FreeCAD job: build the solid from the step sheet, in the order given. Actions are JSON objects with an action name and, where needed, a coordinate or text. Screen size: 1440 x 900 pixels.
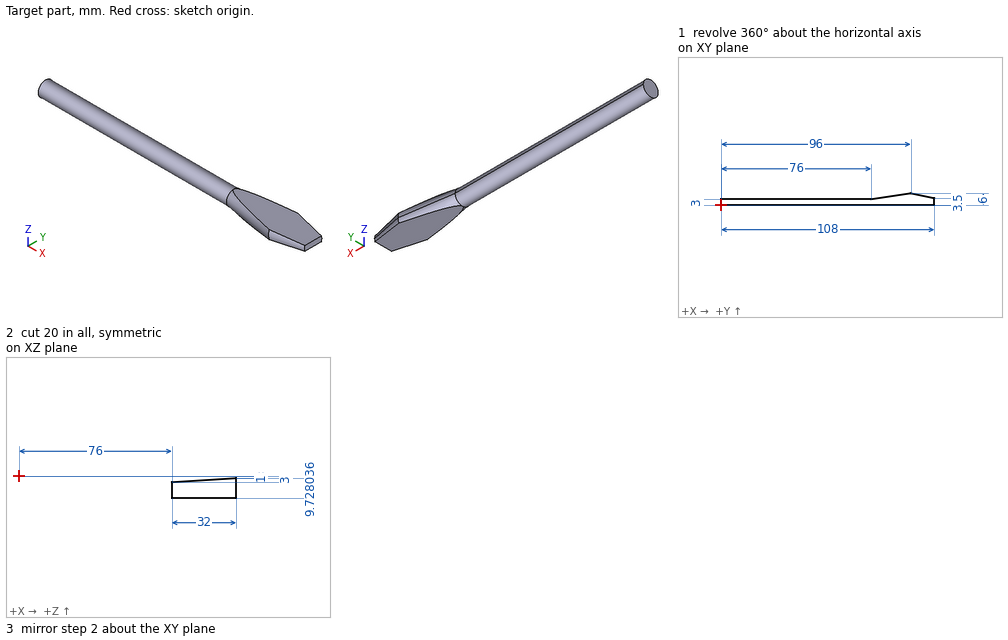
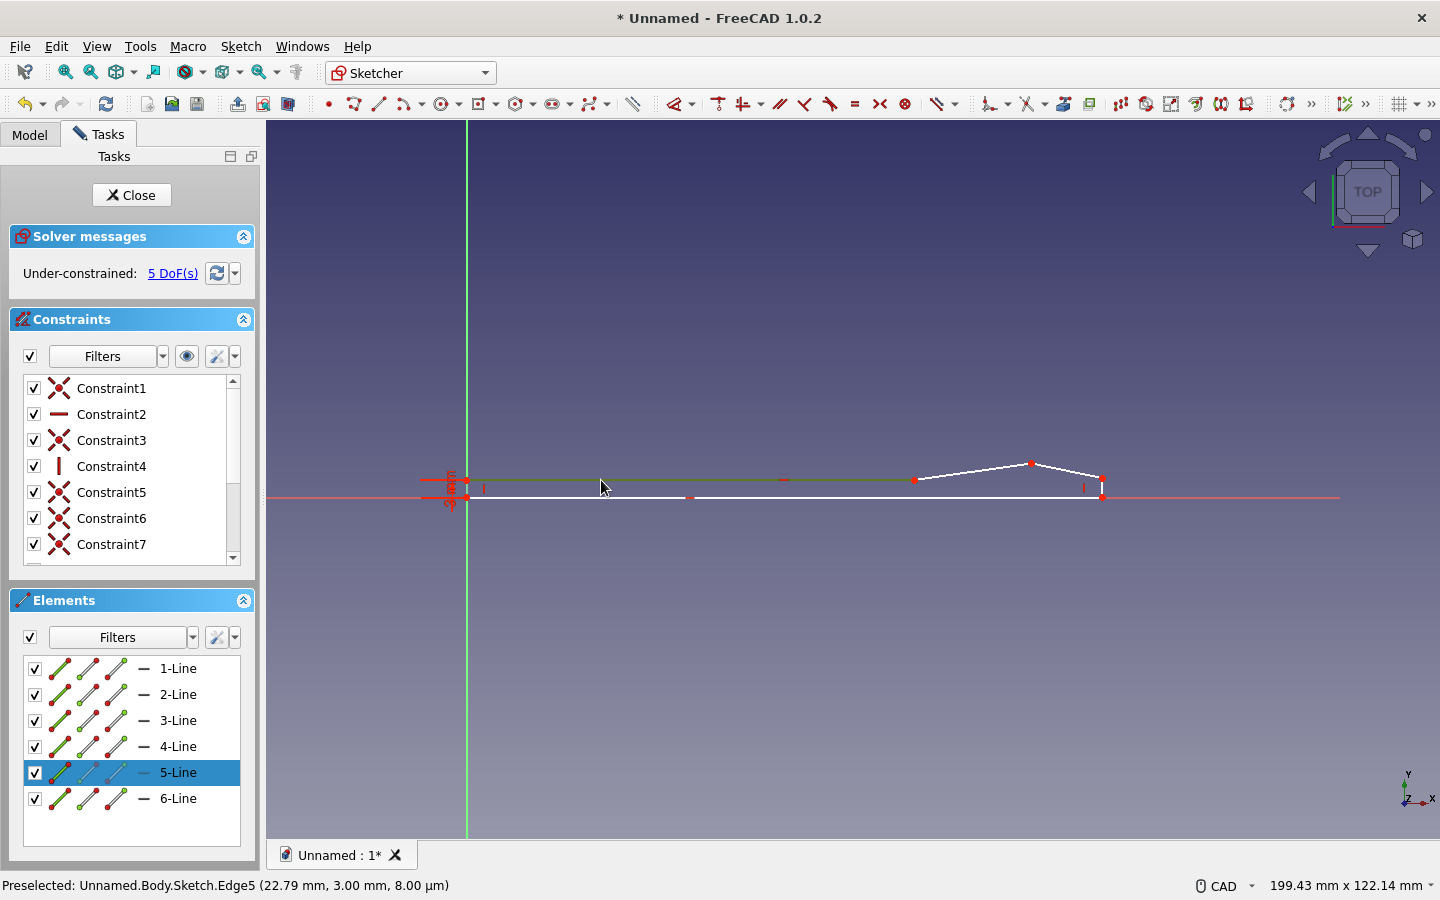
{"action": "key", "text": "l"}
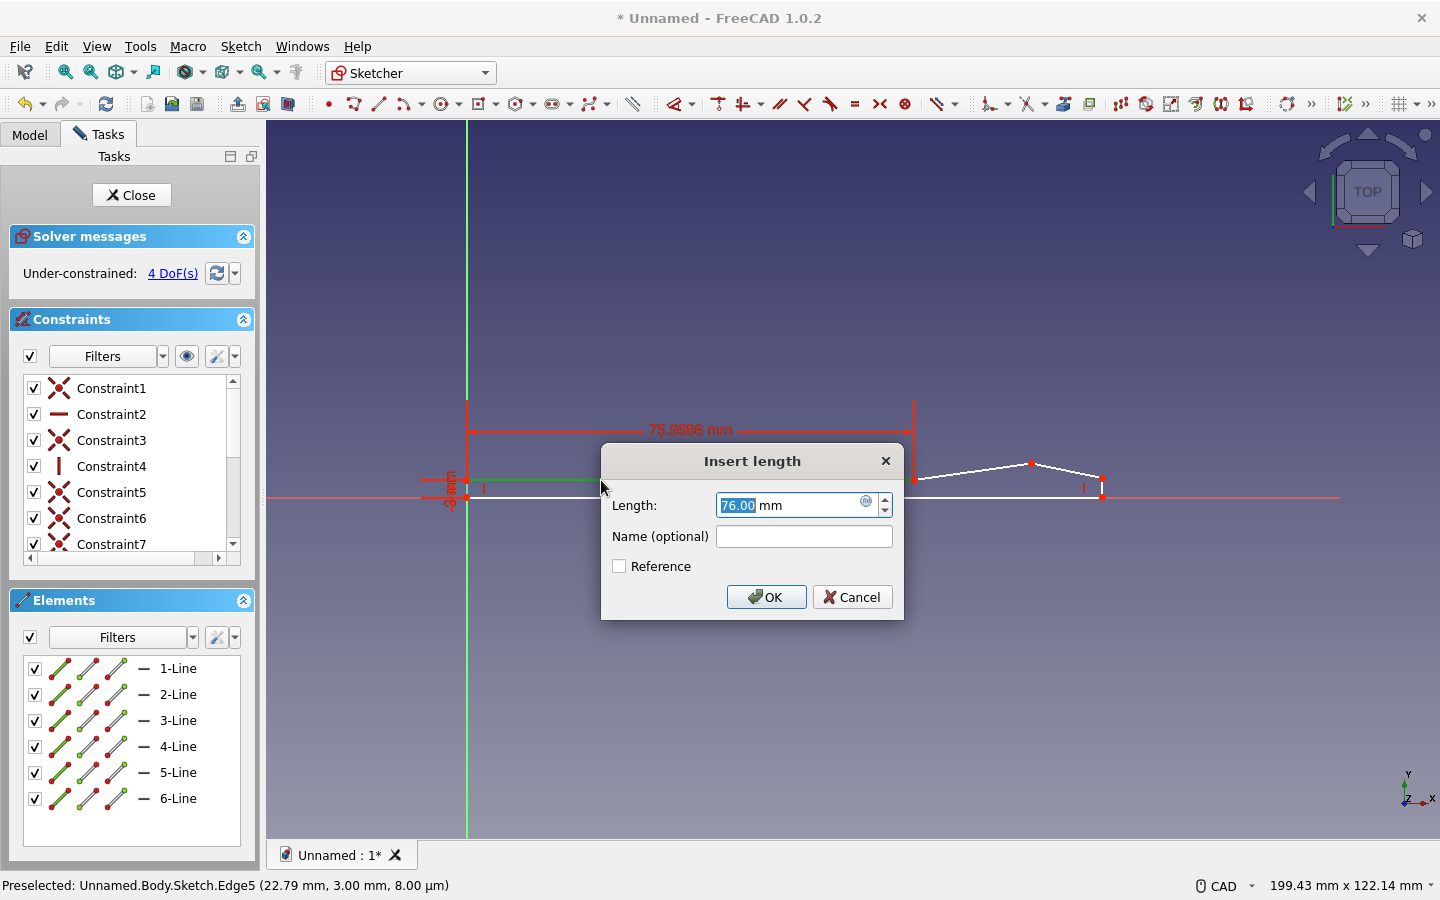
{"action": "type", "text": "76"}
{"action": "key", "text": "Return"}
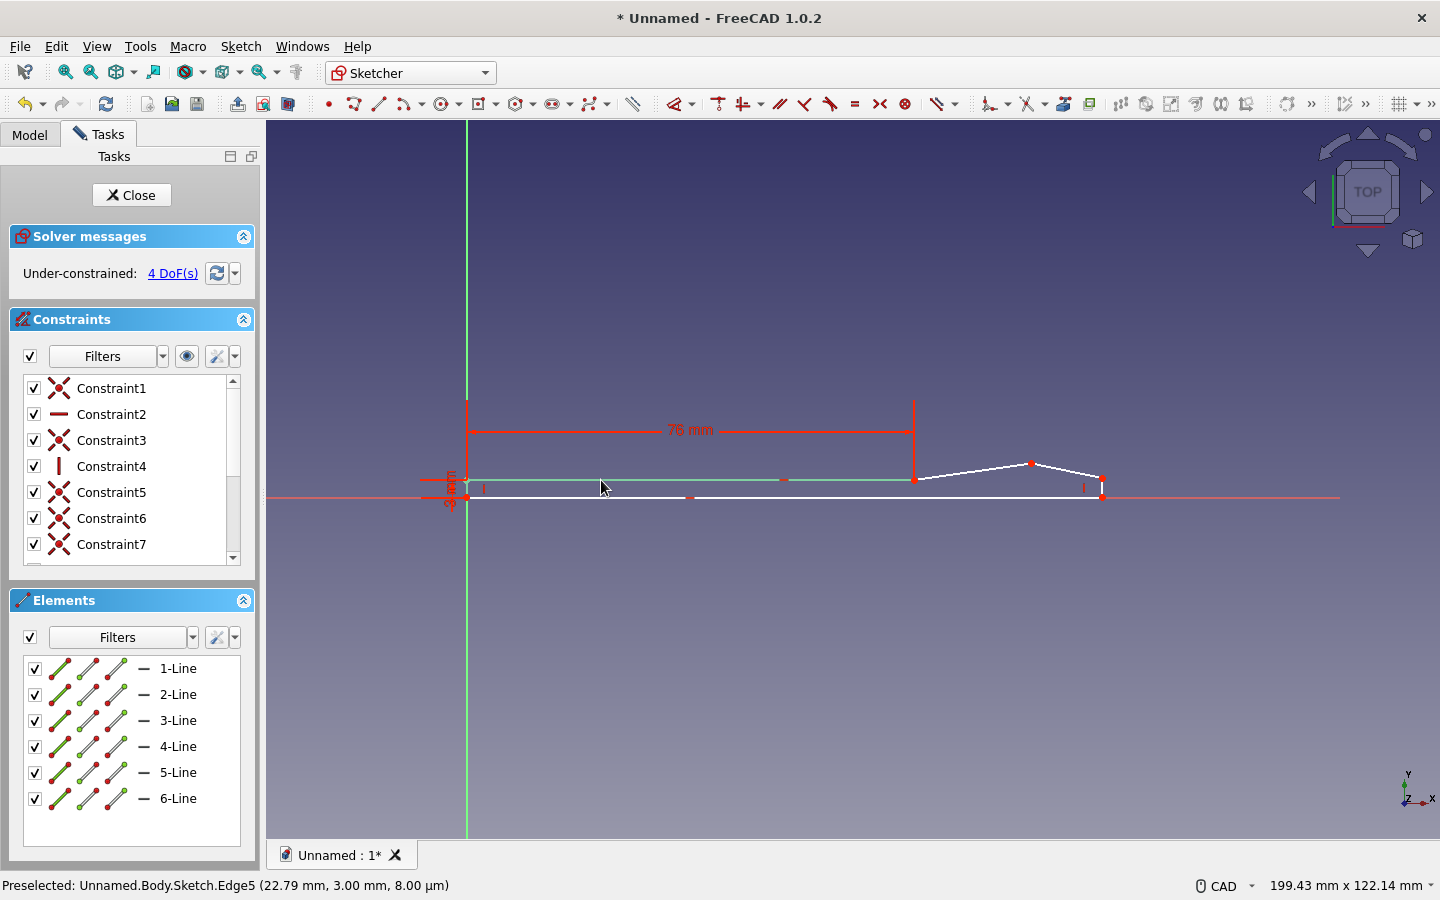
{"action": "left_click", "coordinate": [1032, 463]}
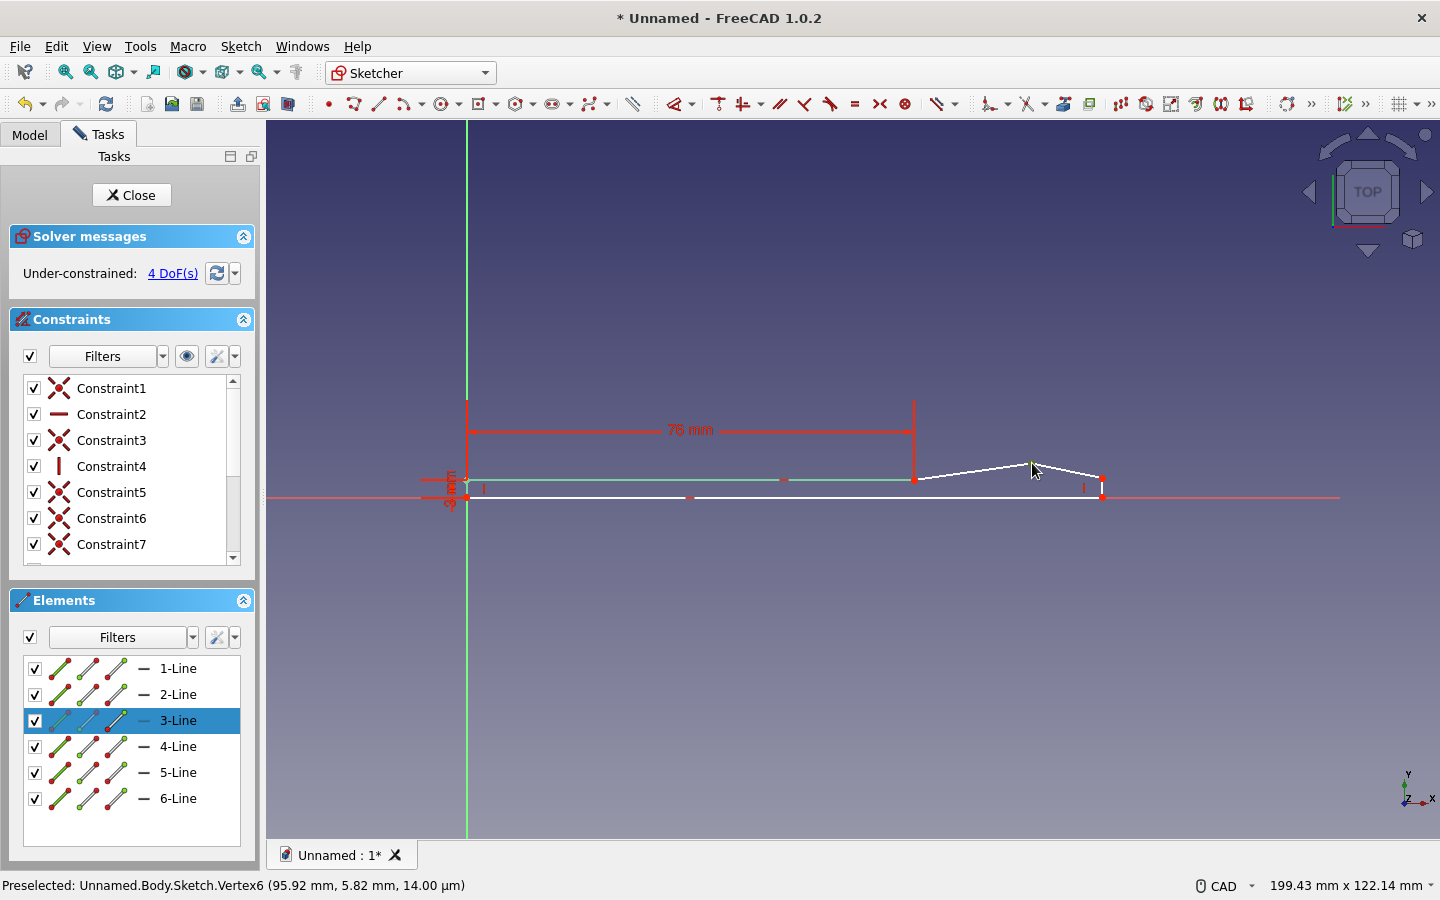
{"action": "key", "text": "i"}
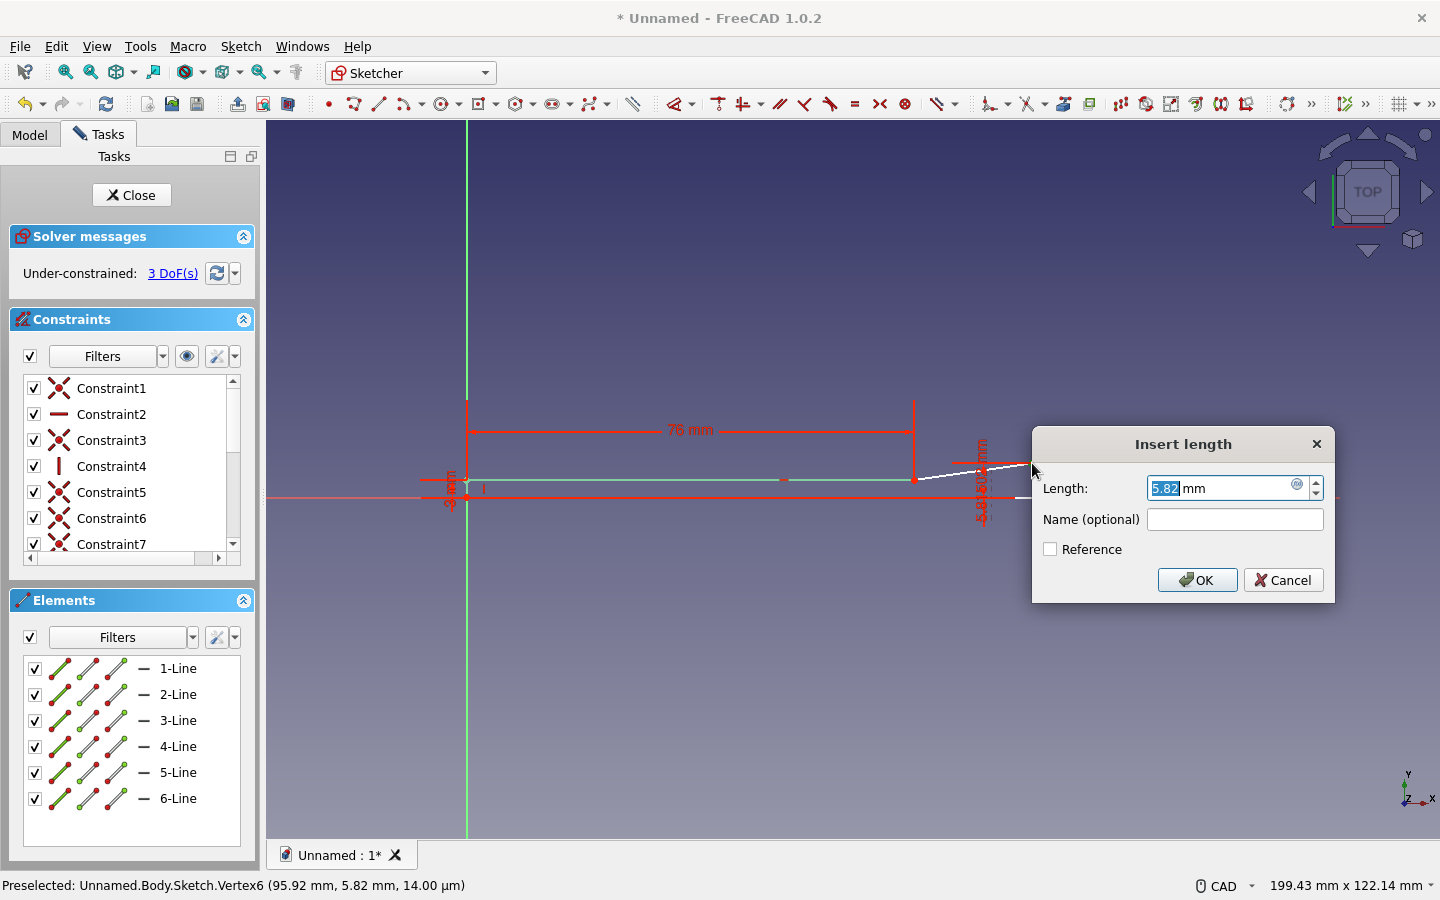
{"action": "type", "text": "6"}
{"action": "key", "text": "Return"}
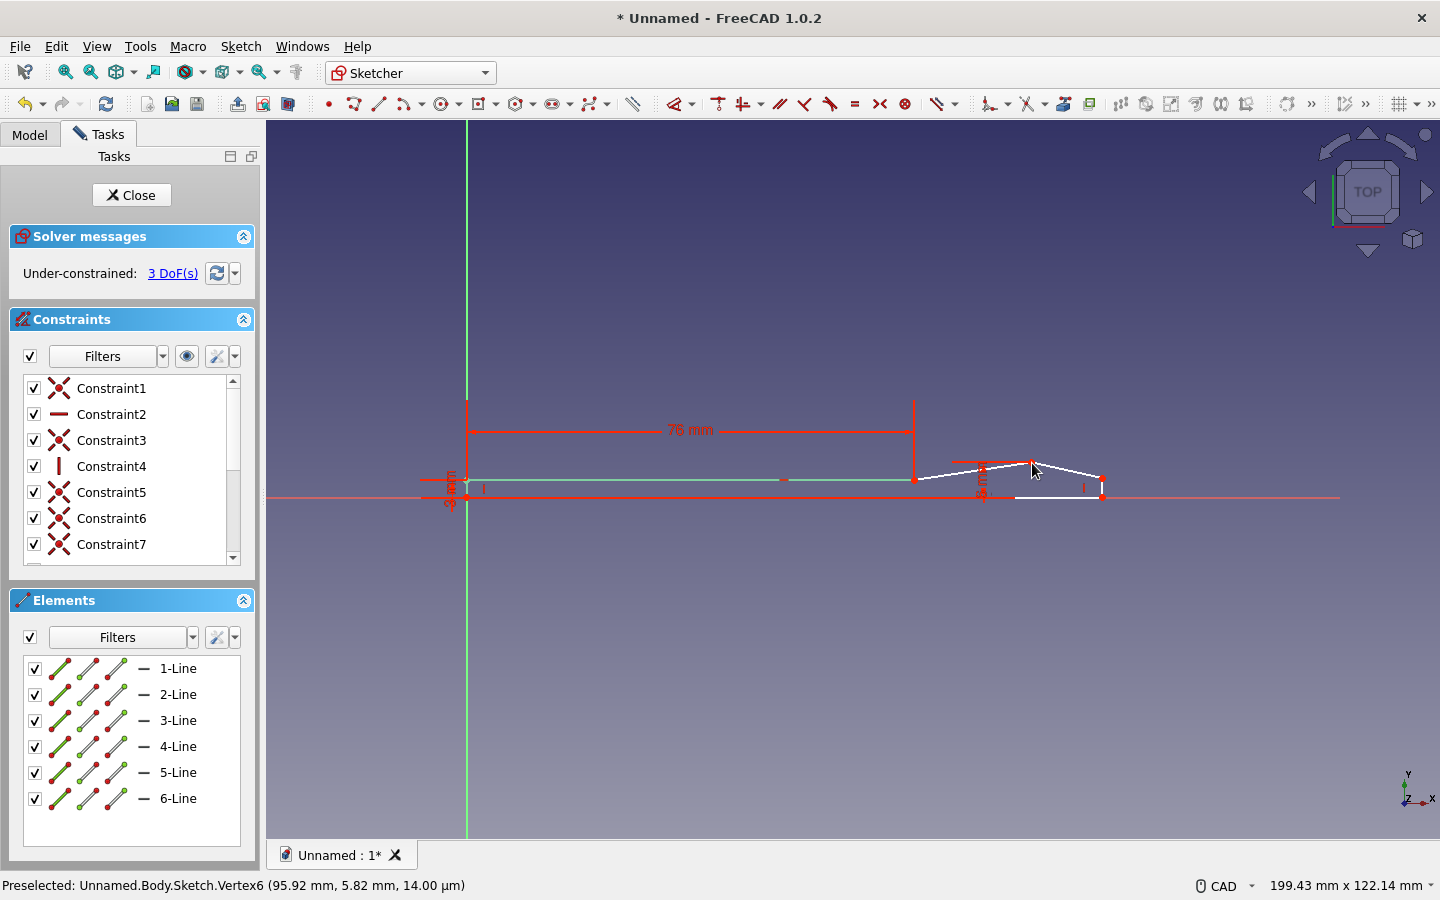
{"action": "left_click", "coordinate": [658, 498]}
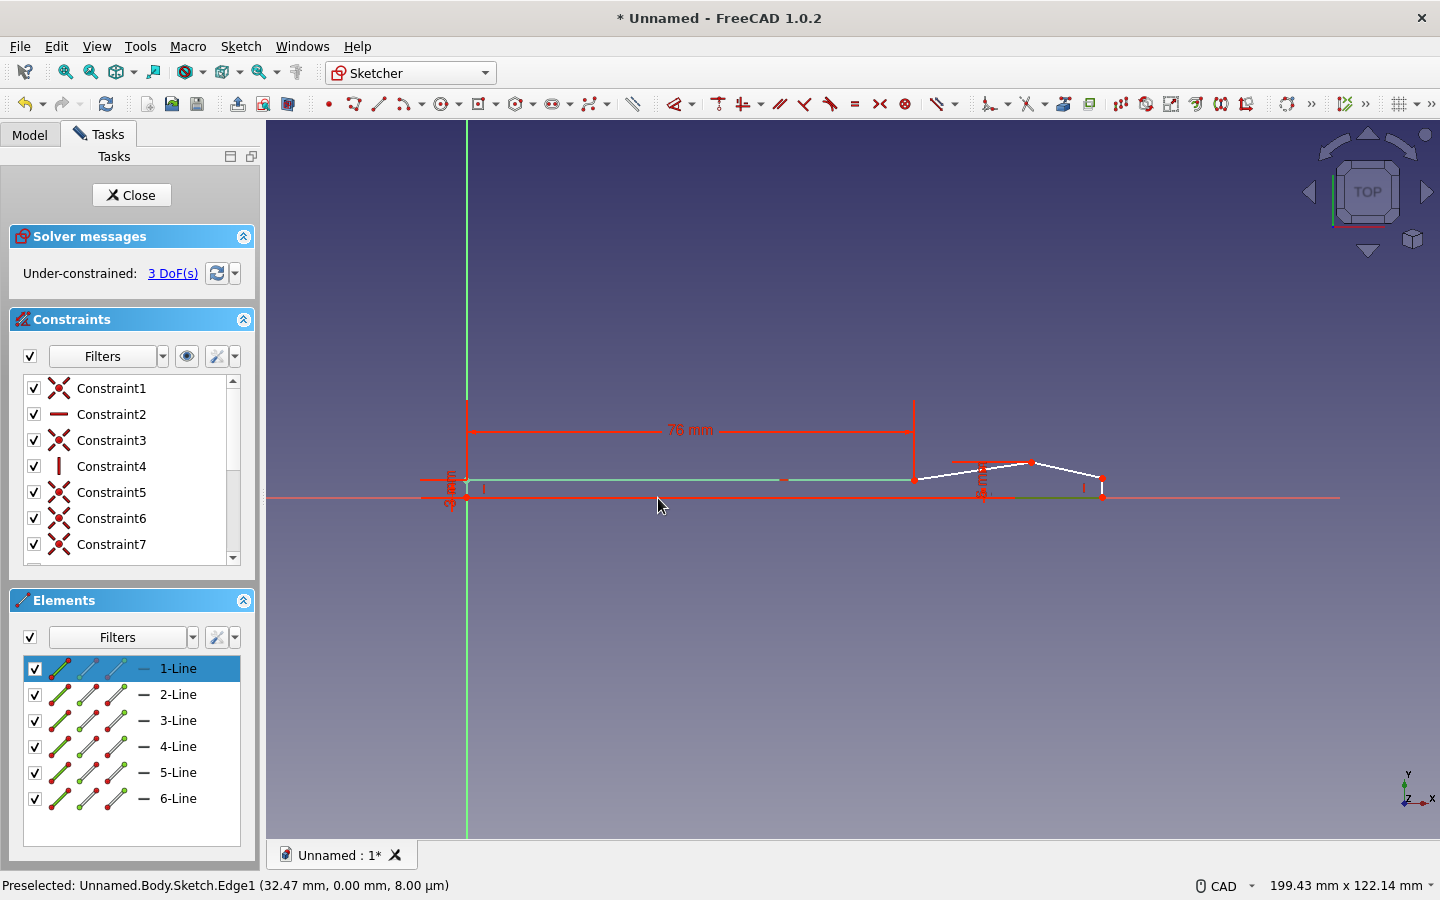
{"action": "left_click", "coordinate": [692, 104]}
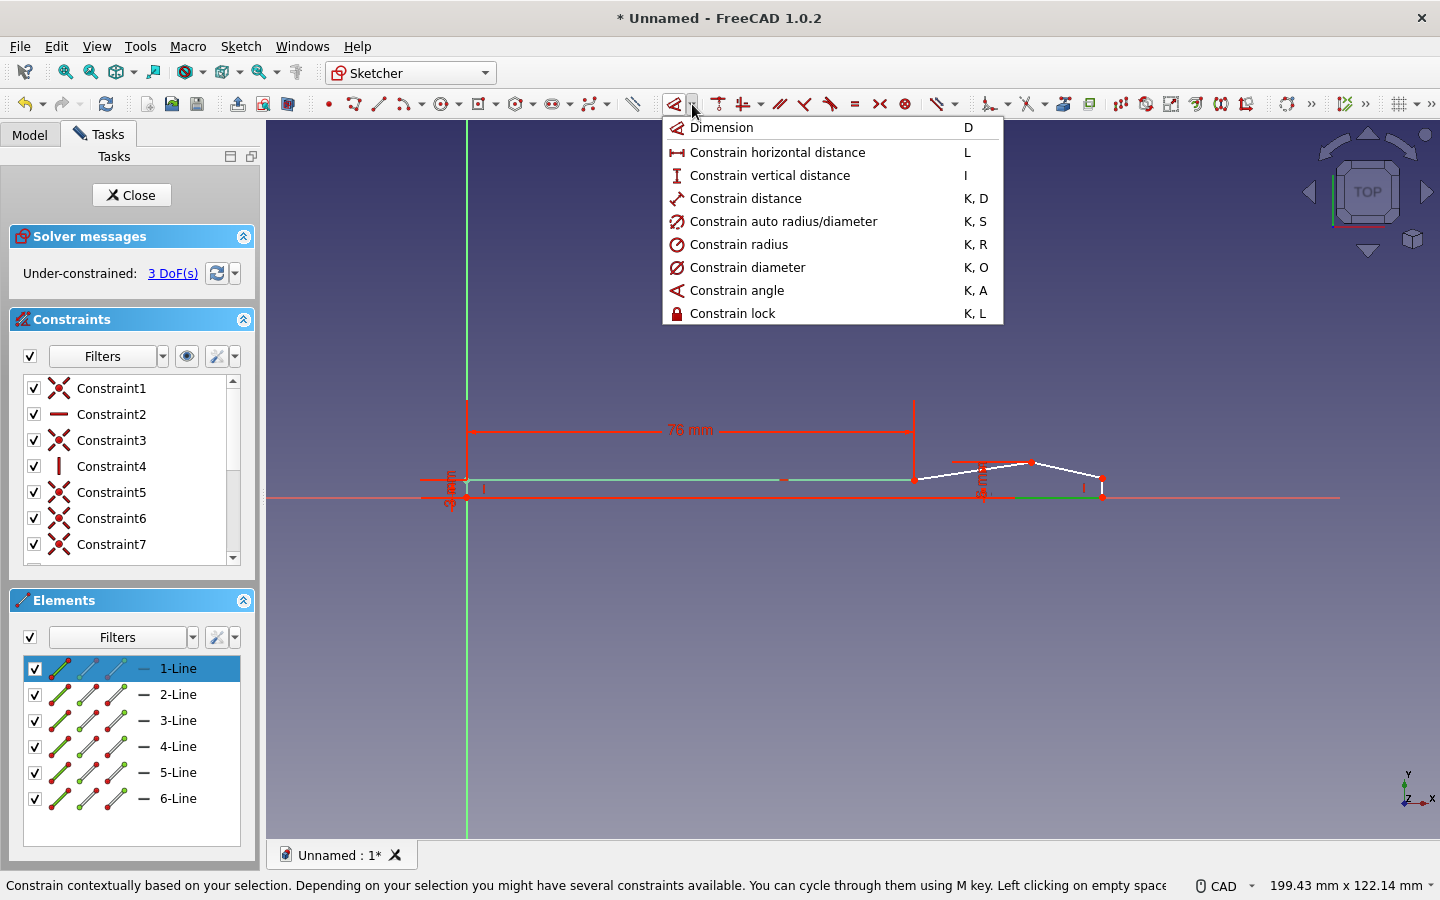
{"action": "left_click", "coordinate": [833, 152]}